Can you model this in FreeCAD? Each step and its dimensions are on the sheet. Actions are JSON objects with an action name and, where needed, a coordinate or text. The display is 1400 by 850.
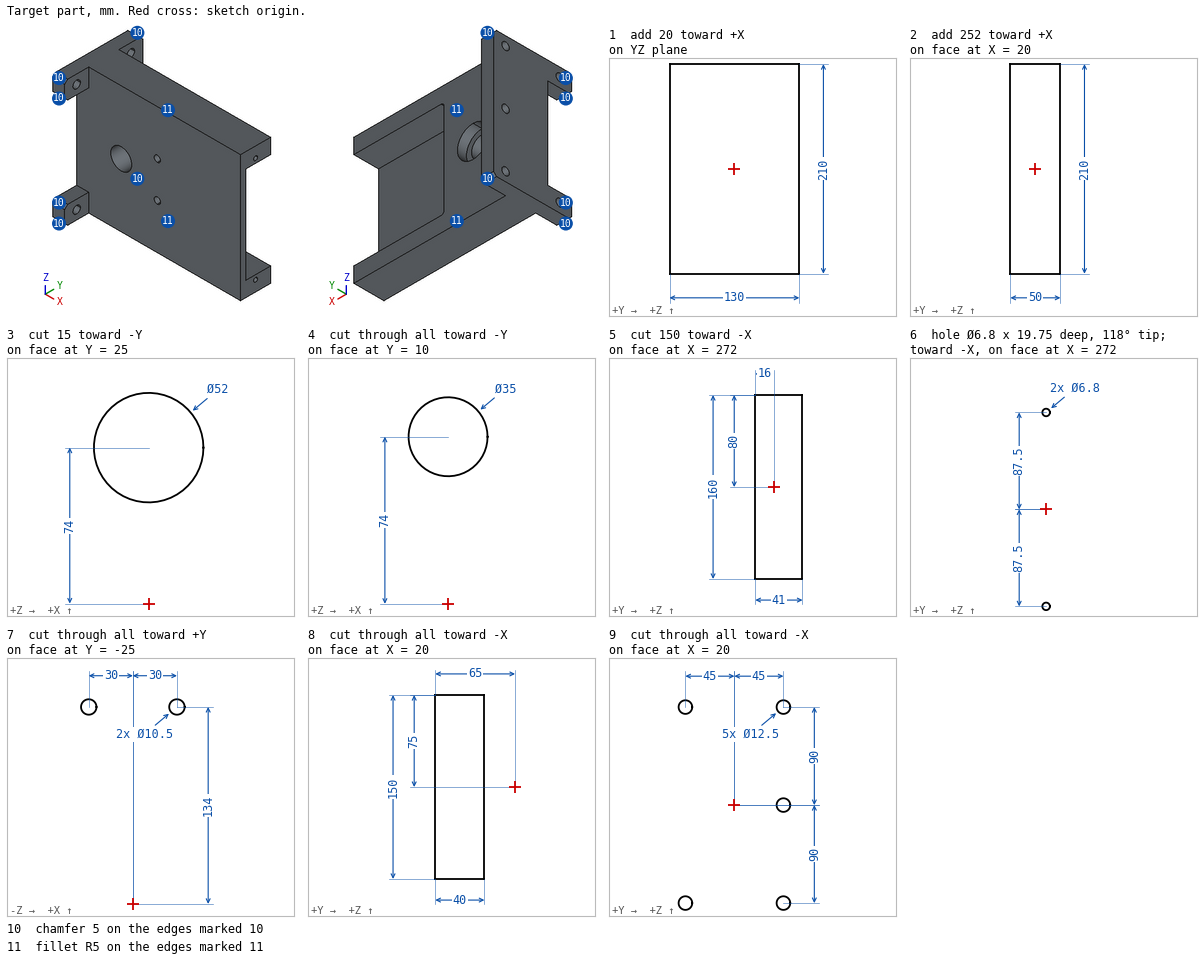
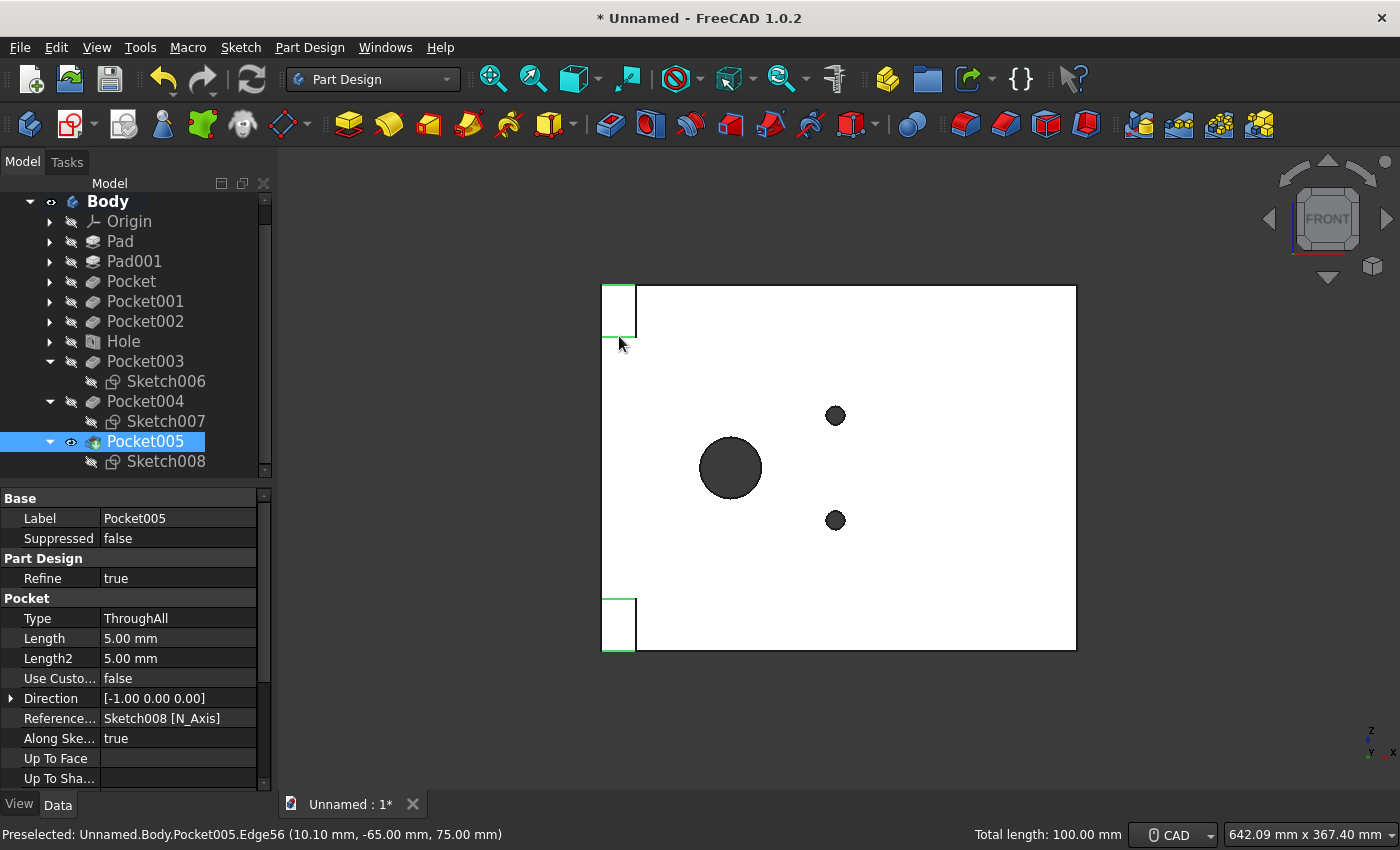
{"action": "key", "text": "3"}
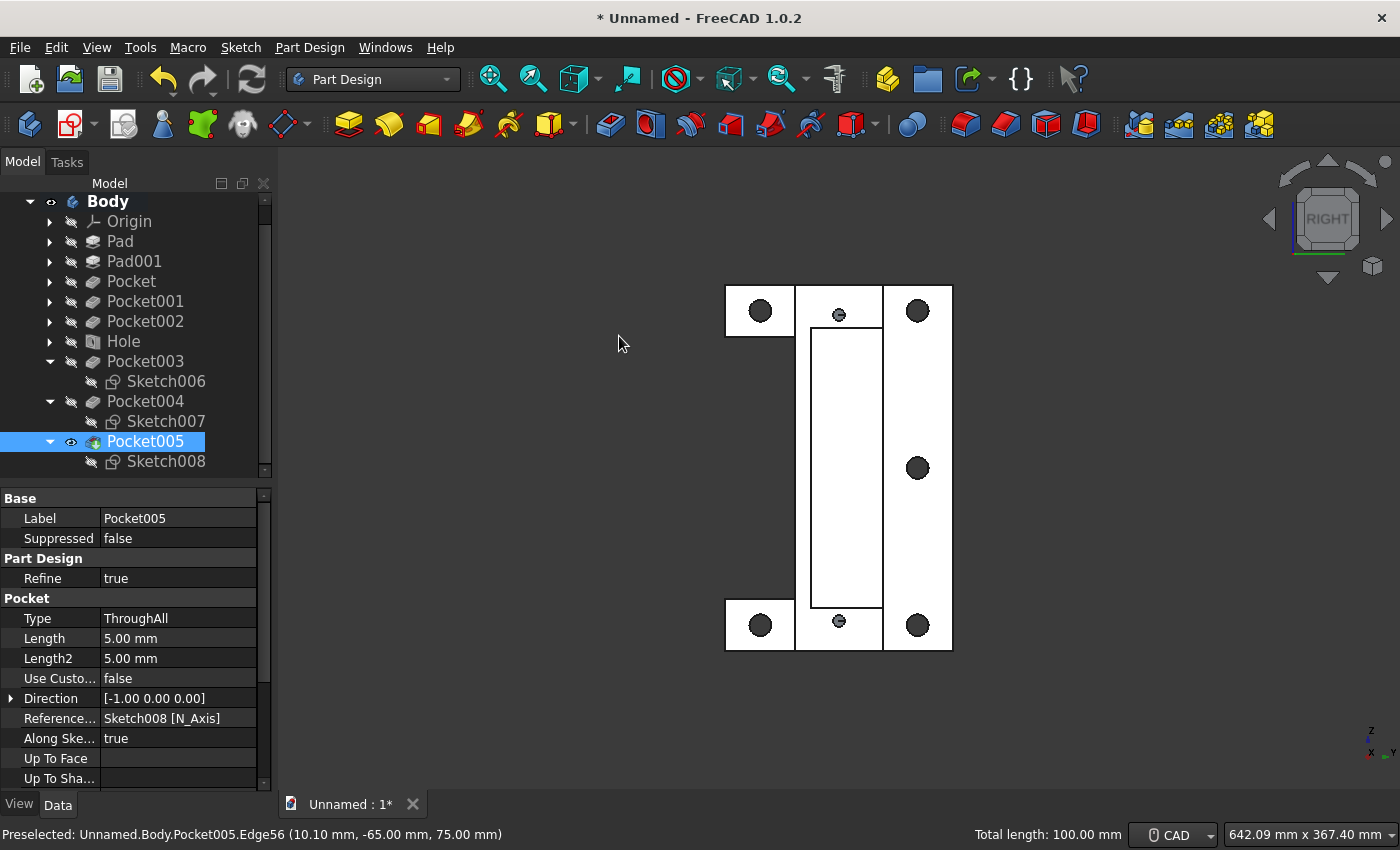
{"action": "key", "text": "5"}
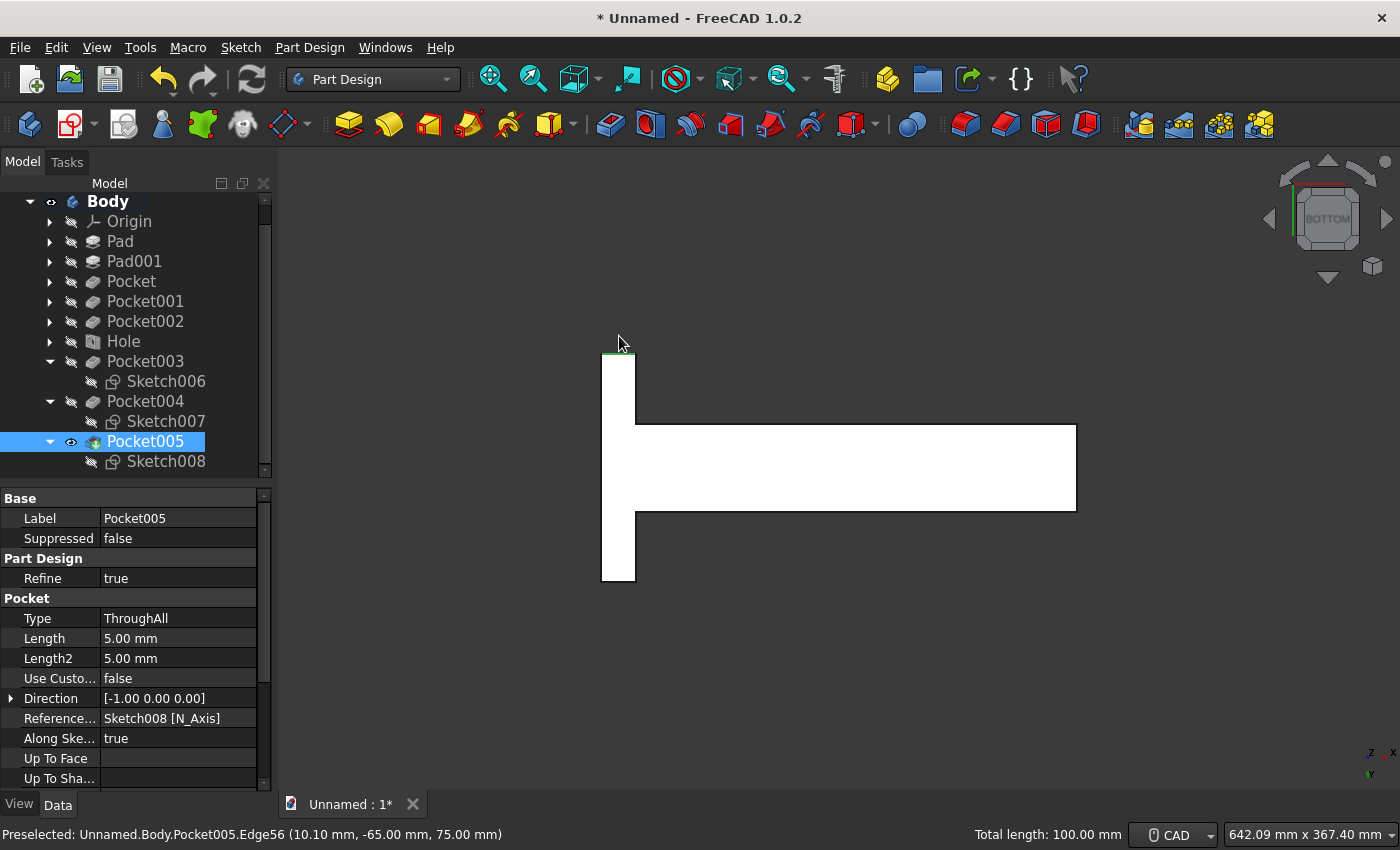
{"action": "left_click", "coordinate": [494, 80]}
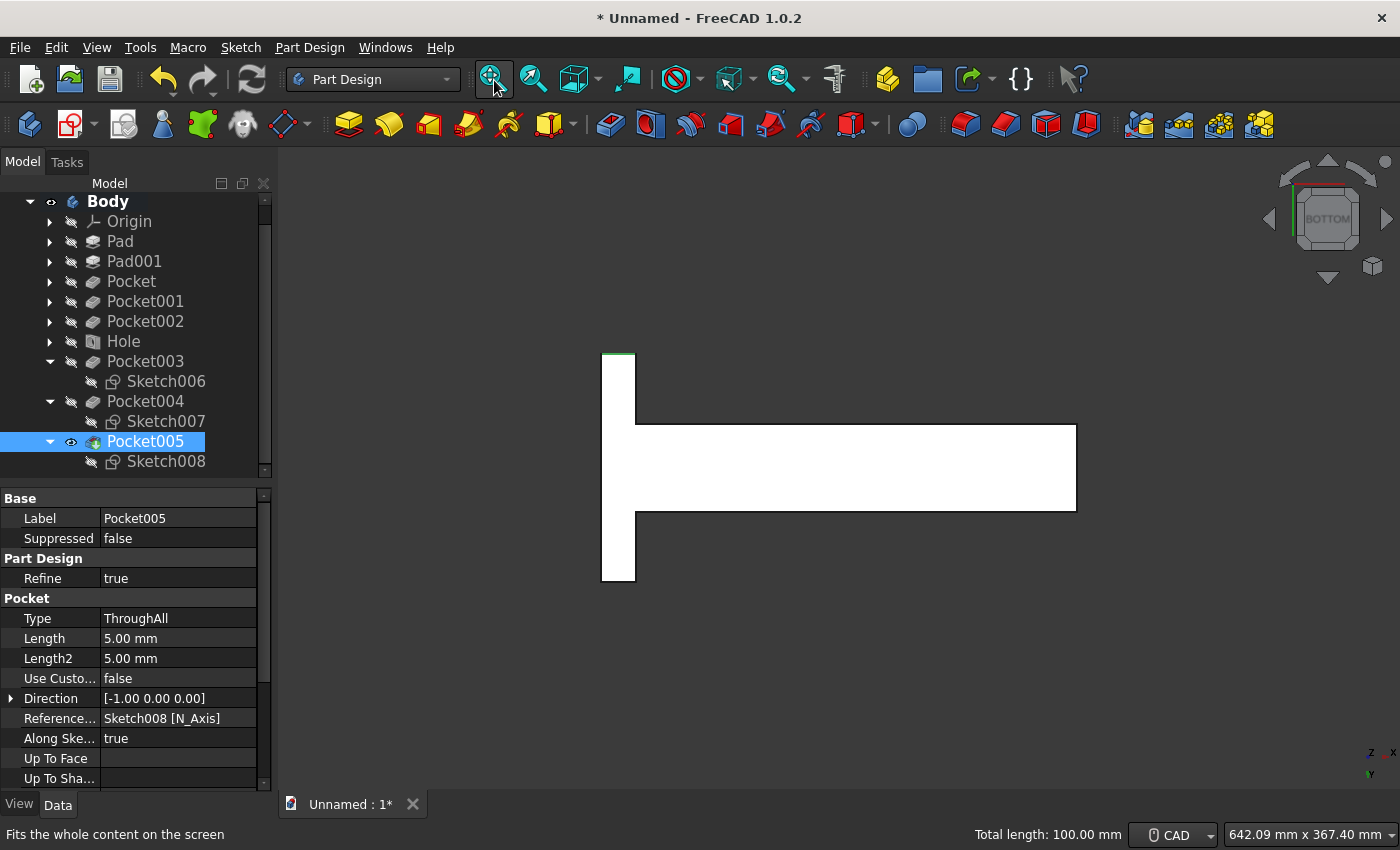
{"action": "left_click", "coordinate": [619, 581], "text": "ctrl"}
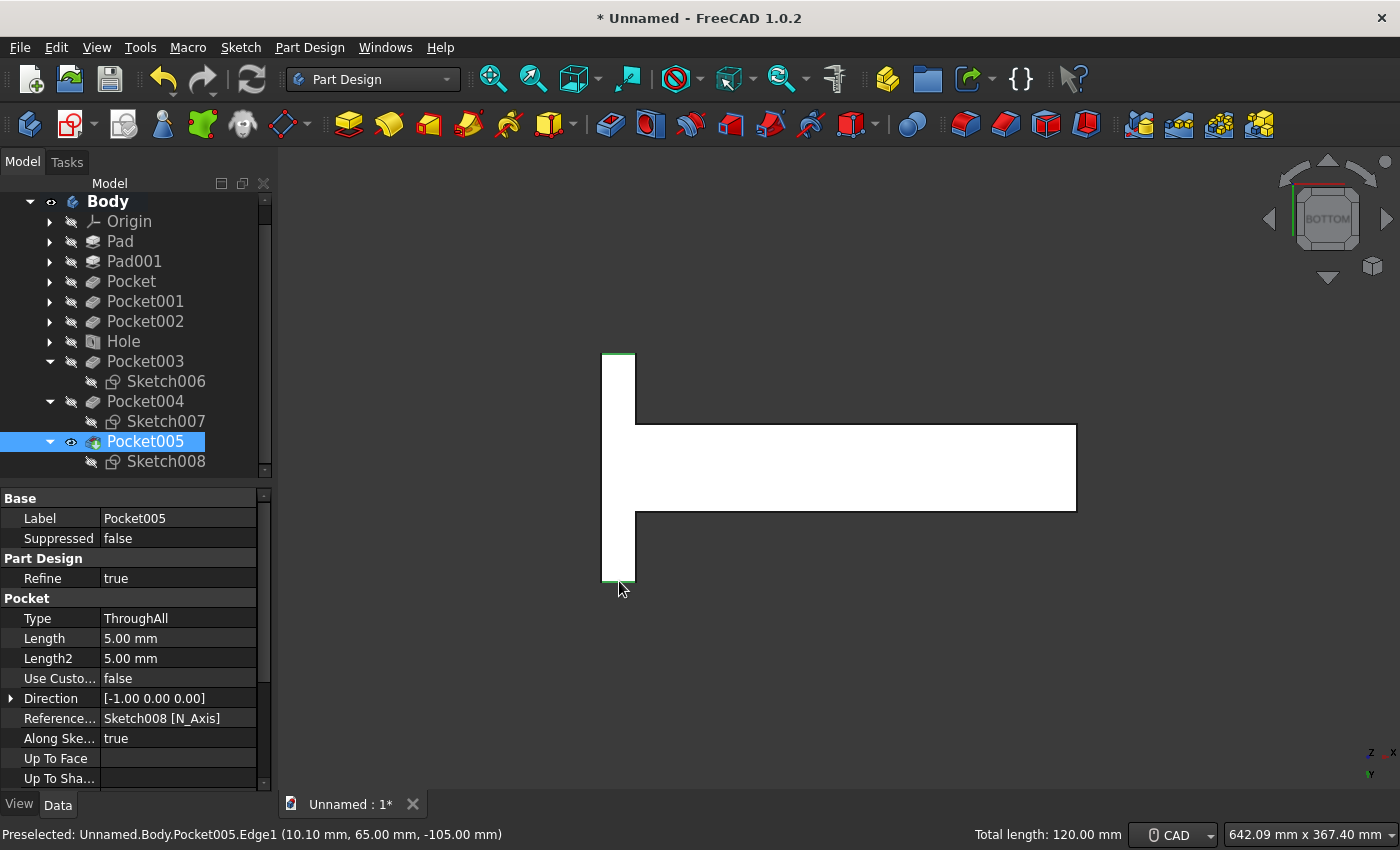
{"action": "left_click", "coordinate": [1006, 124]}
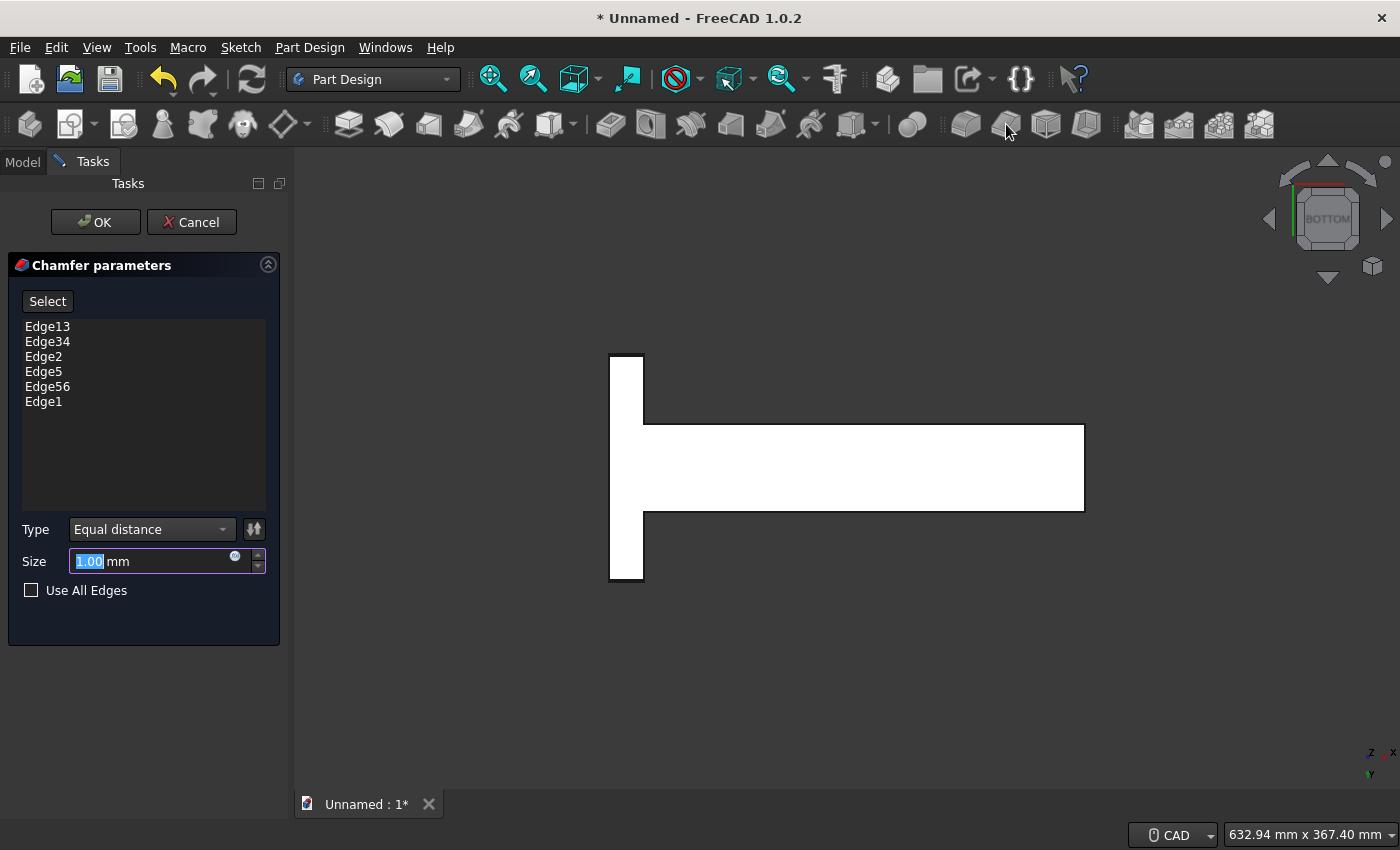
{"action": "type", "text": "5"}
{"action": "key", "text": "Tab"}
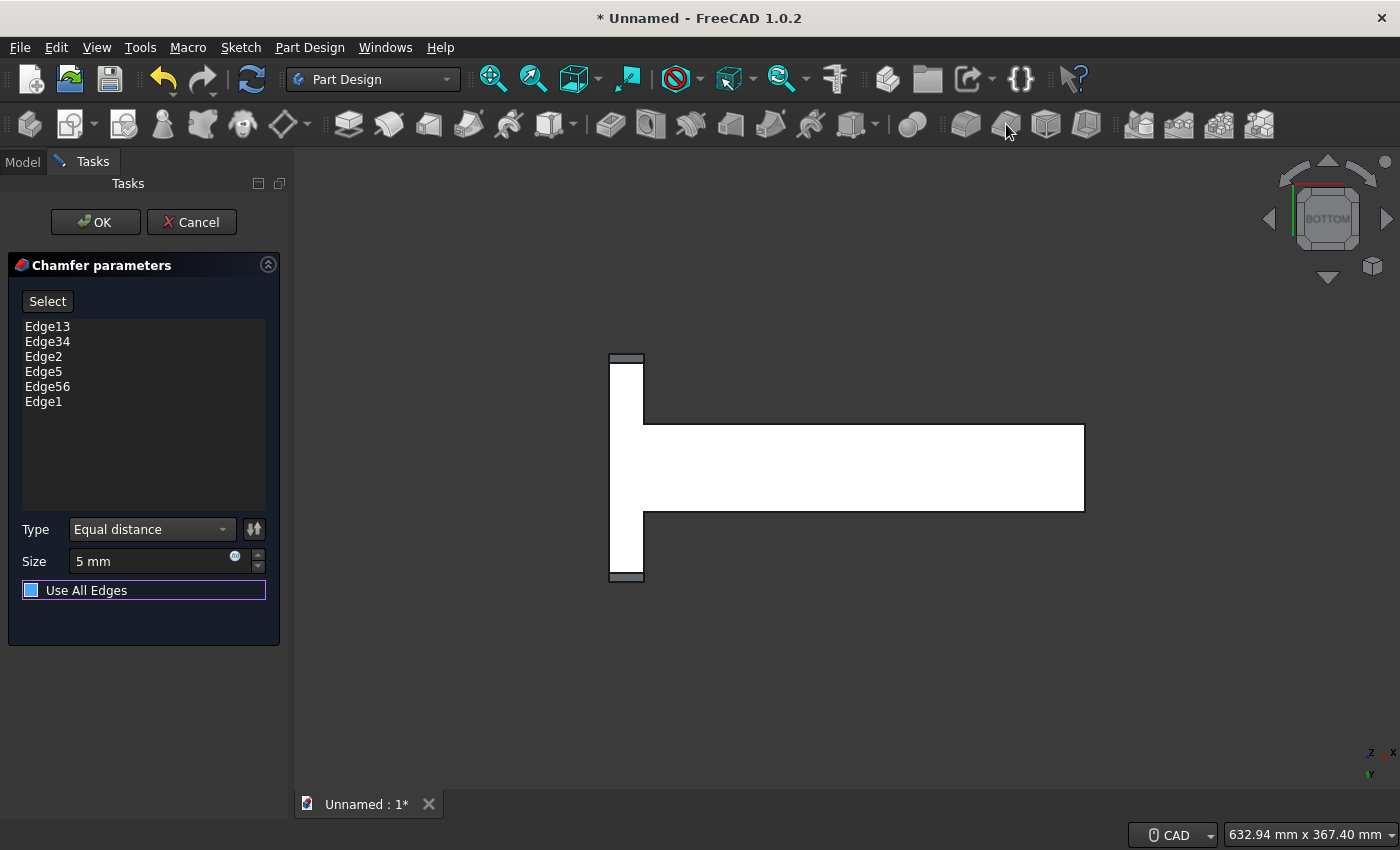
{"action": "left_click", "coordinate": [96, 222]}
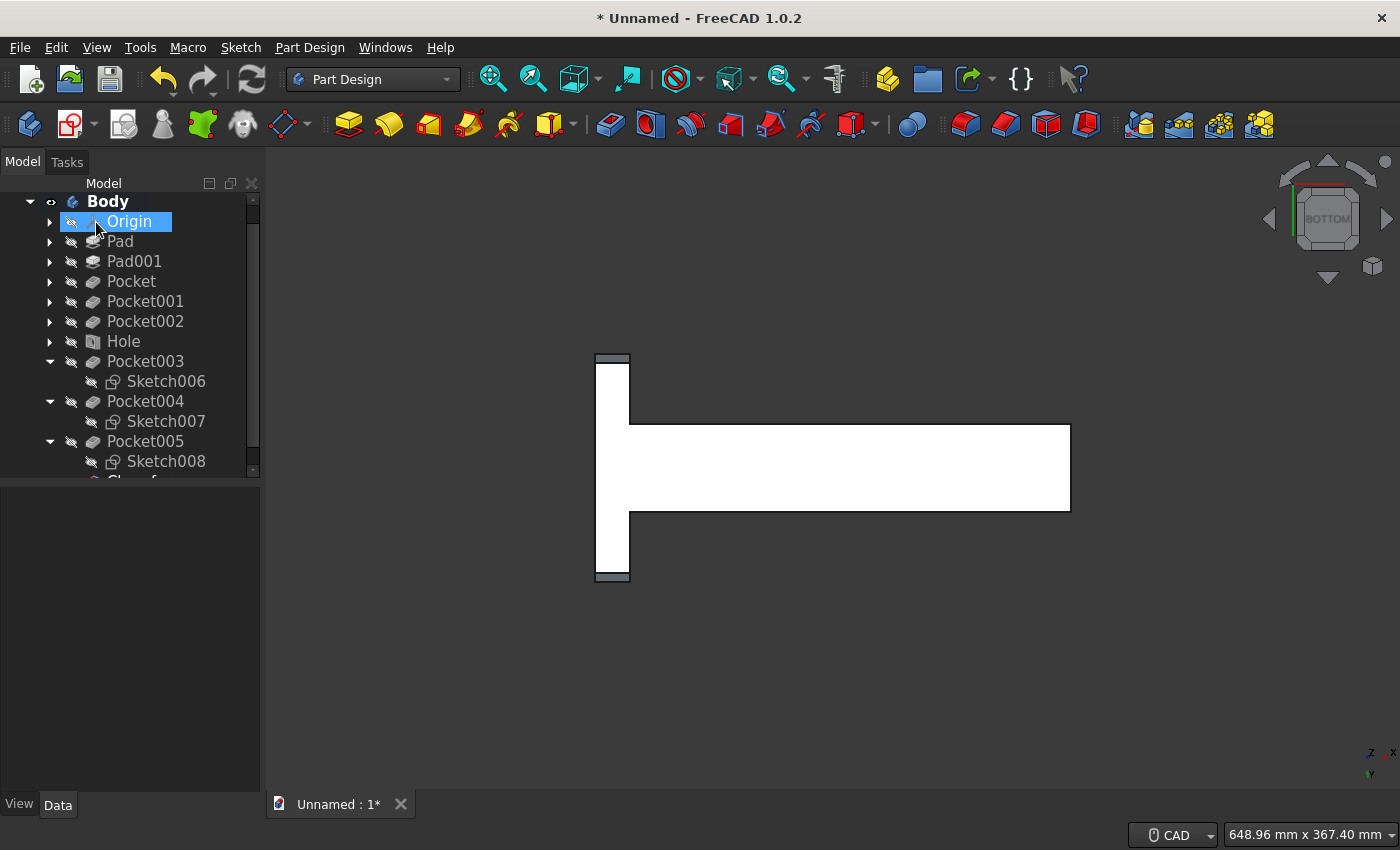
{"action": "left_click", "coordinate": [494, 80]}